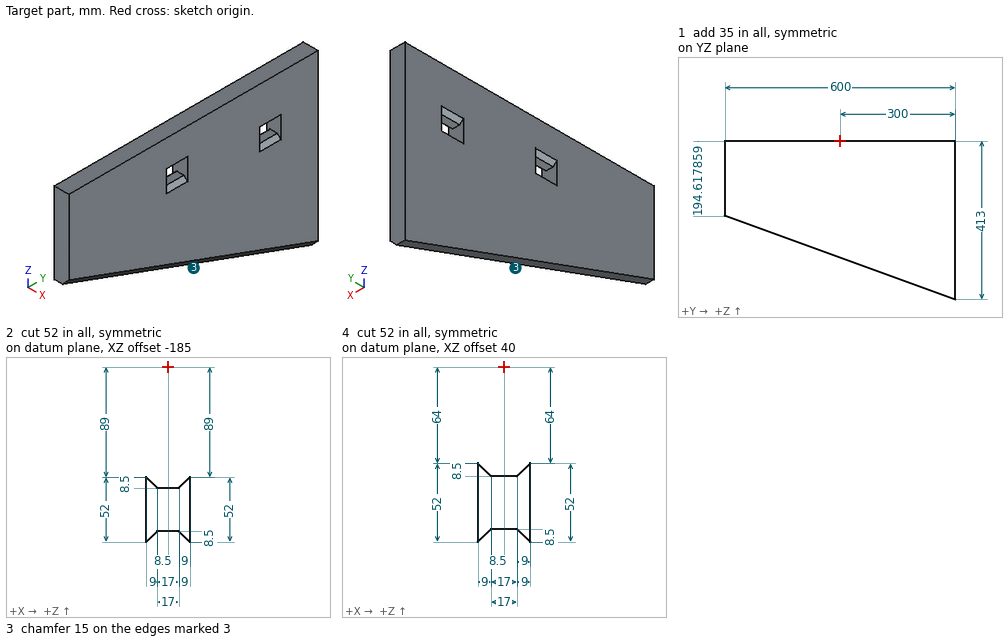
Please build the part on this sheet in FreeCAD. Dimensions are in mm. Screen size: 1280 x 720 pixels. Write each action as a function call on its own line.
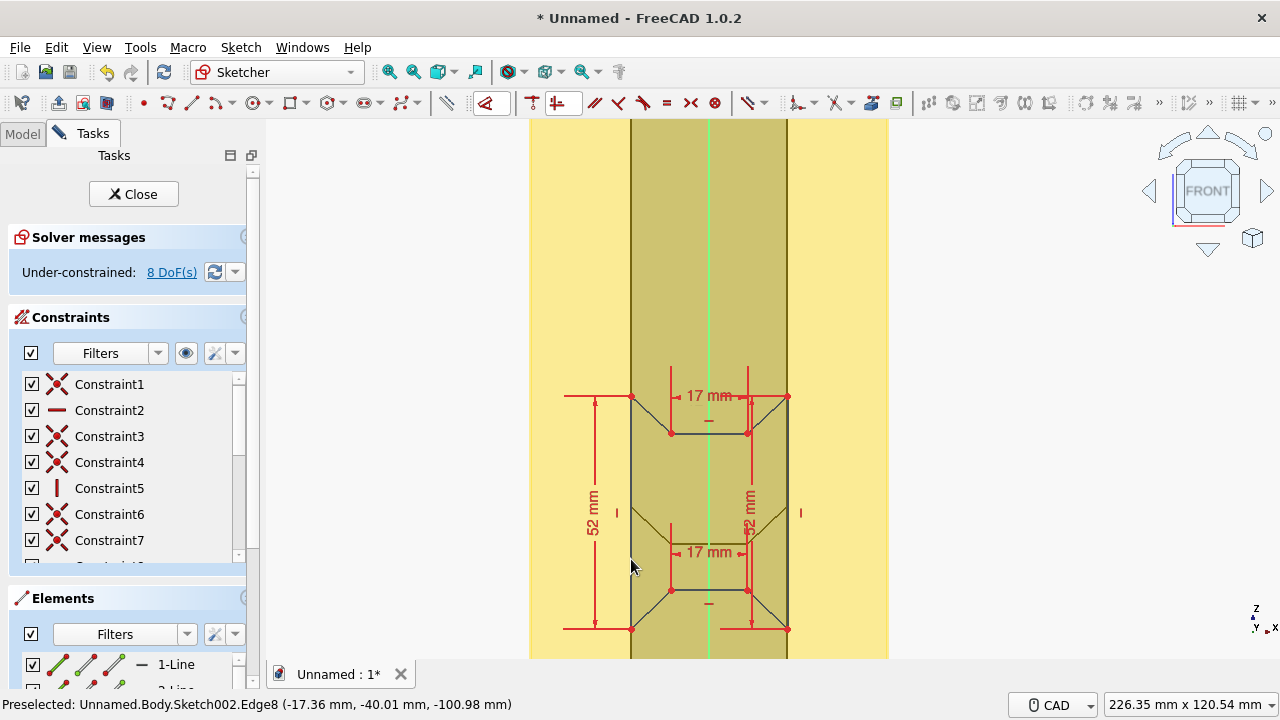
click(643, 408)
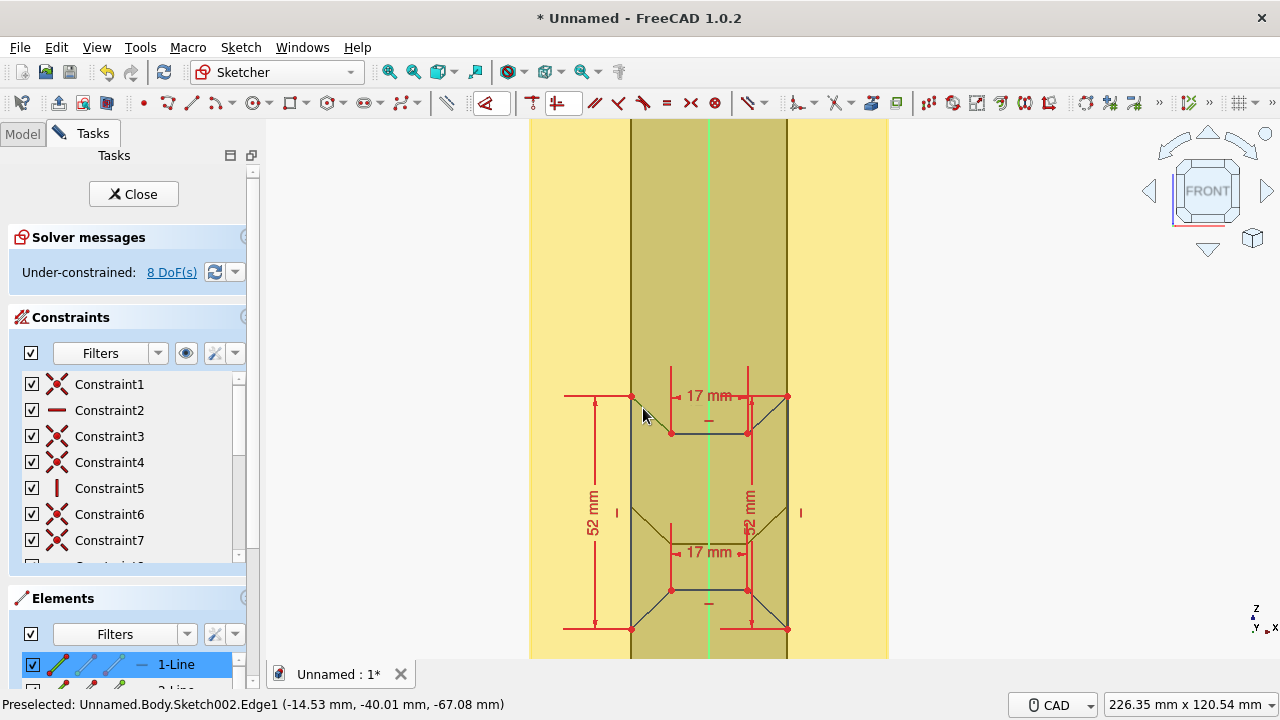
key(l)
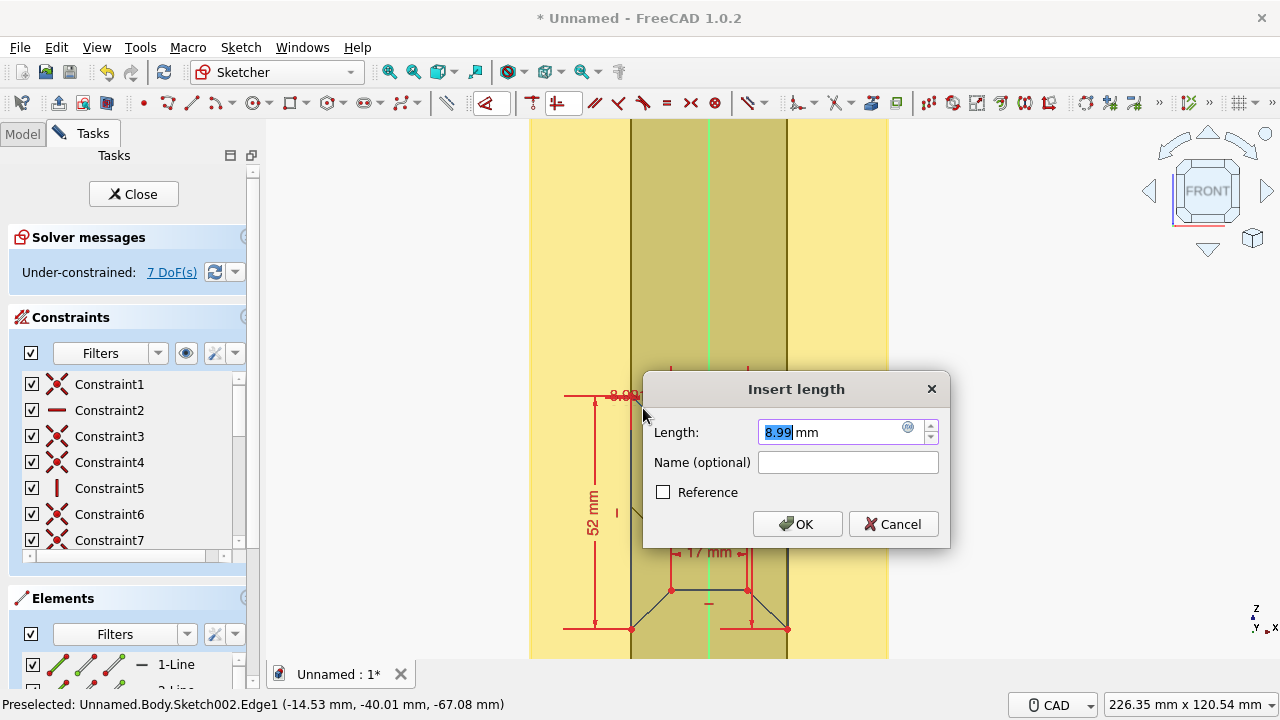
text(9)
key(Return)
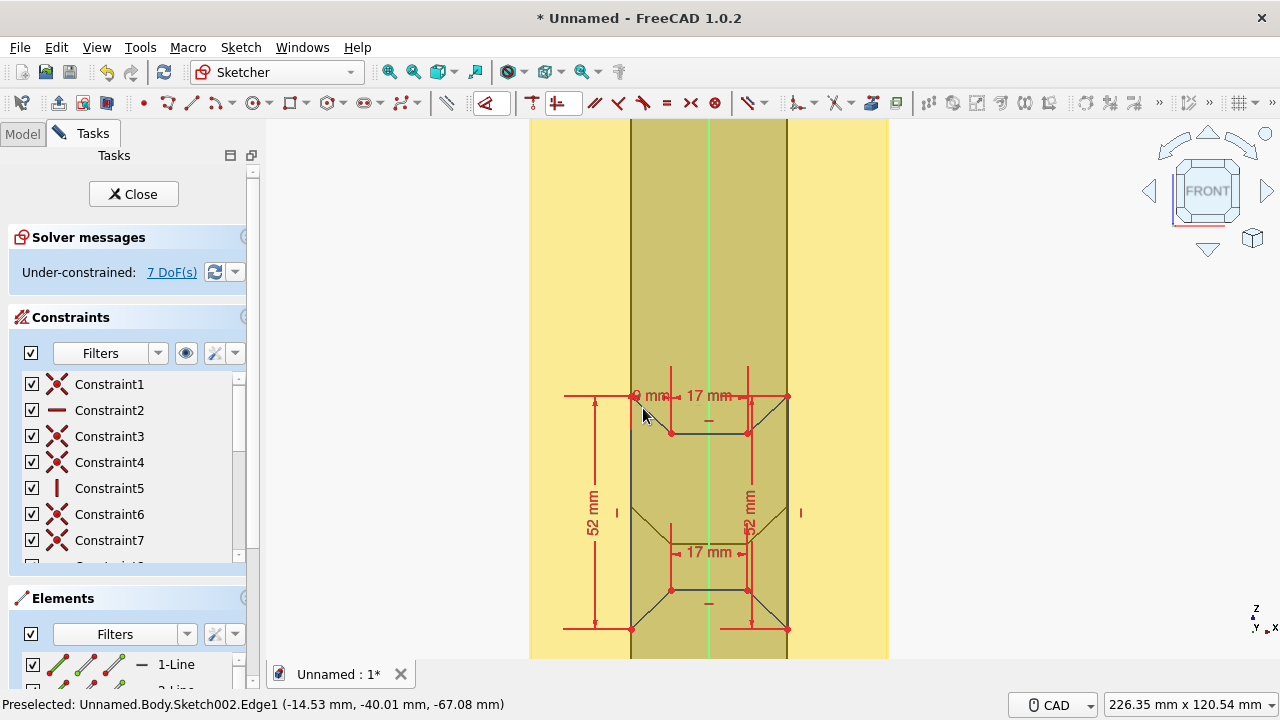
click(760, 422)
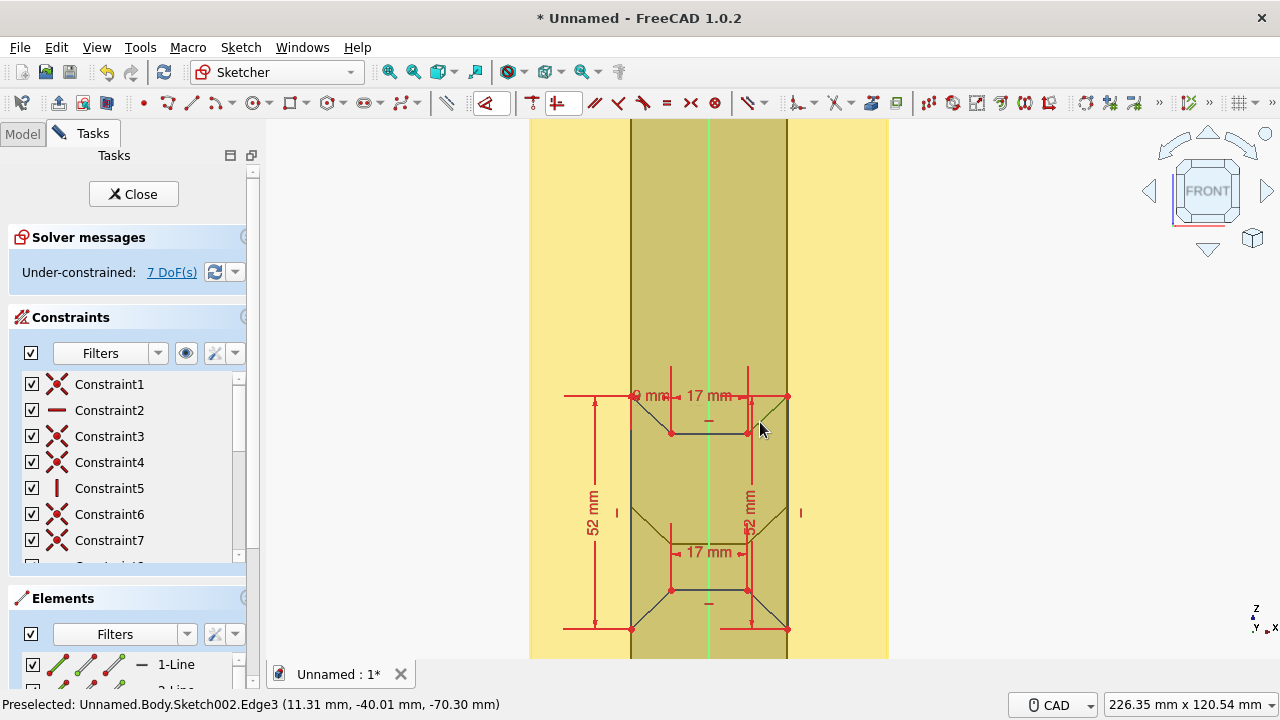
click(504, 104)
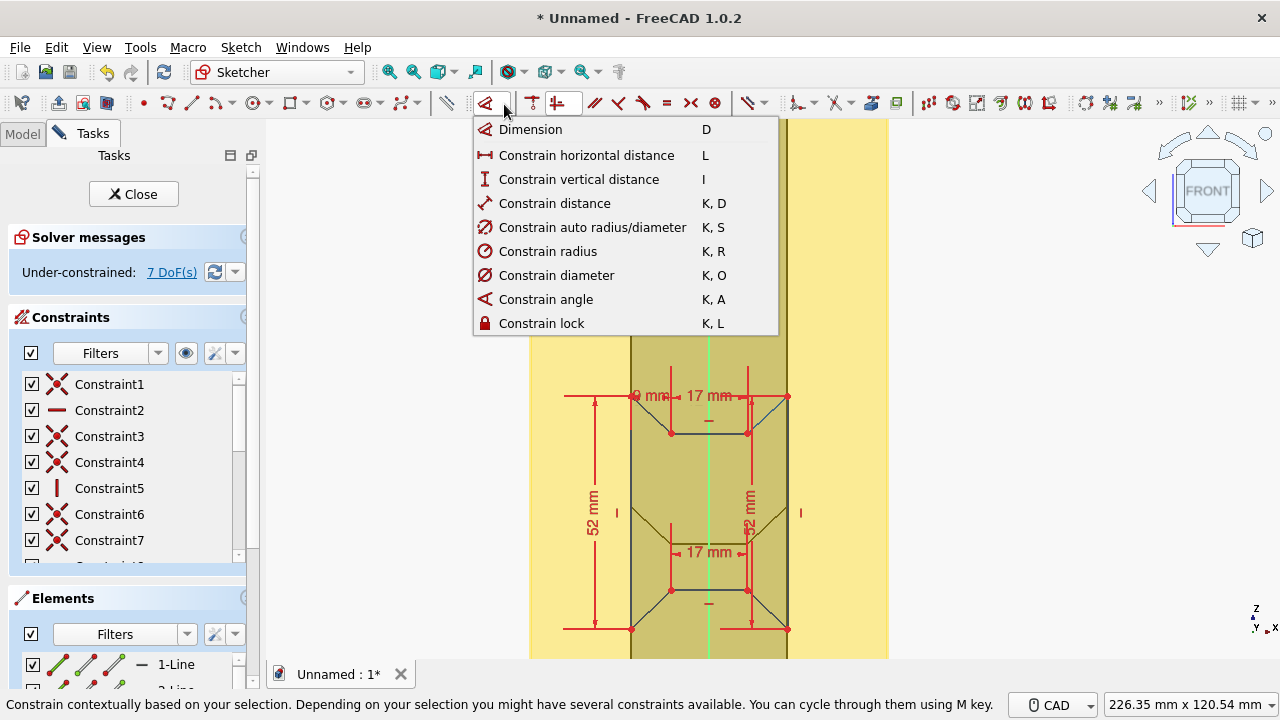
click(626, 155)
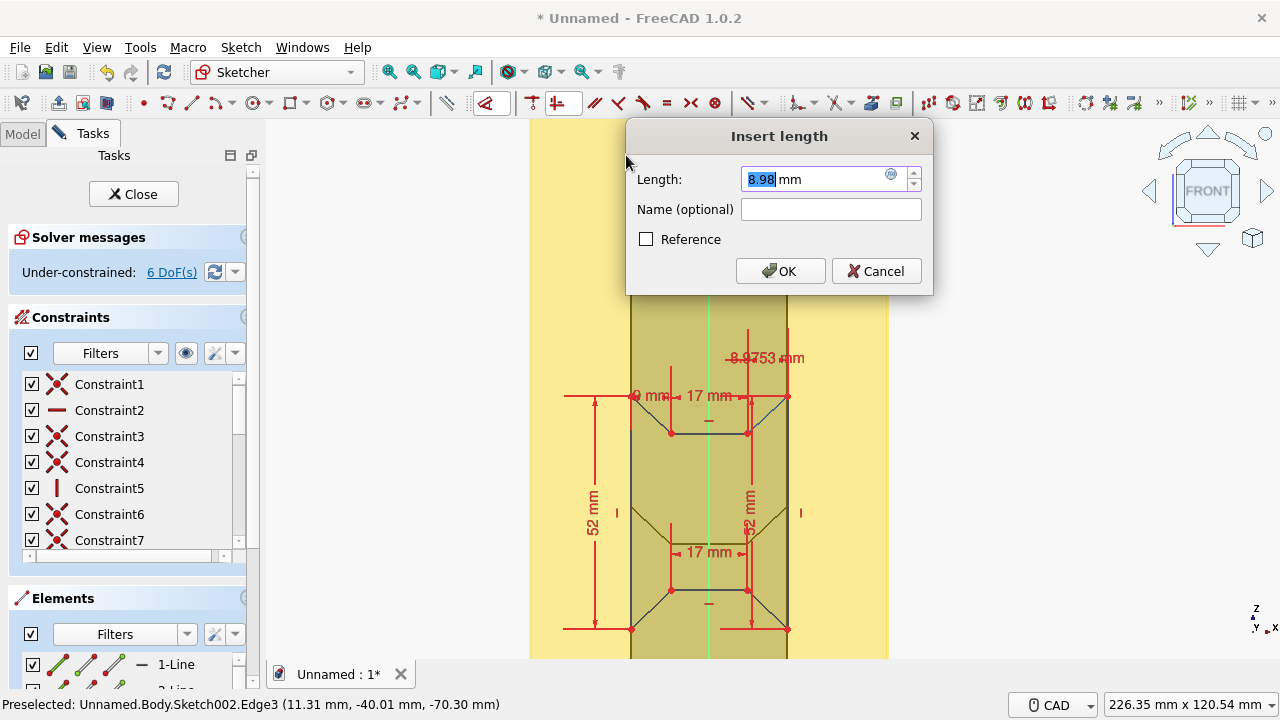
text(9)
key(Return)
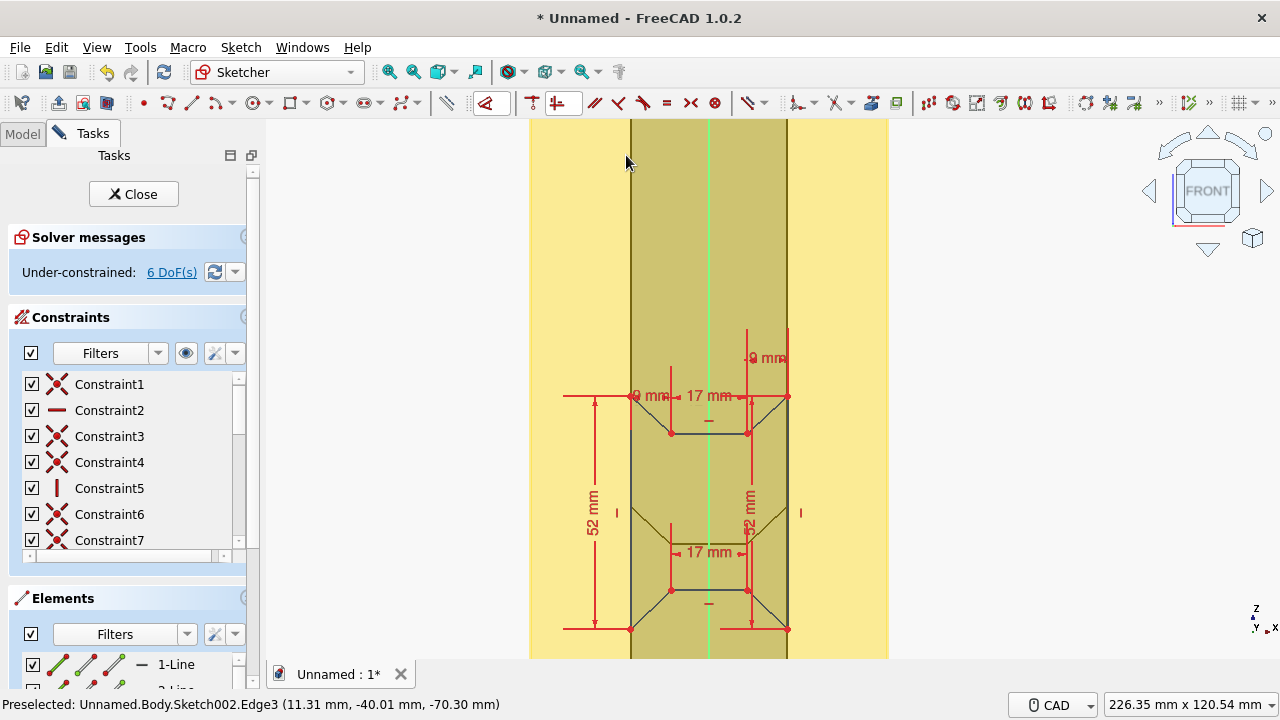
click(776, 618)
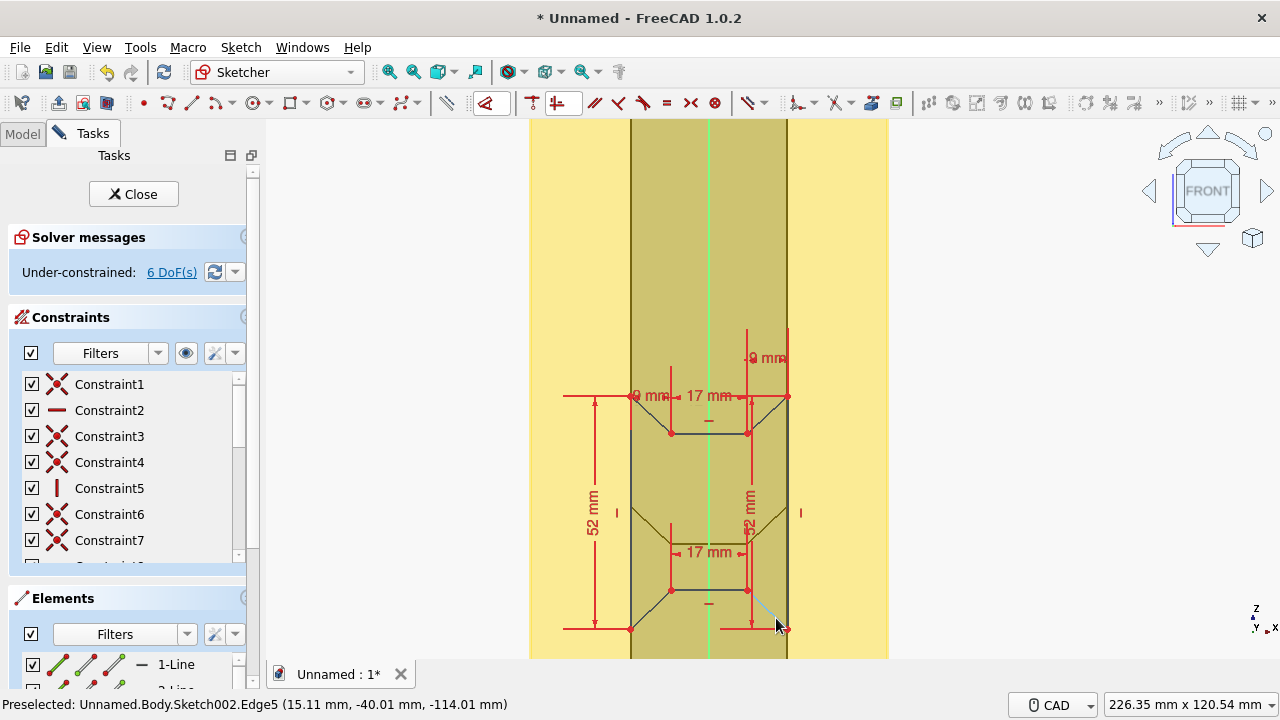
key(l)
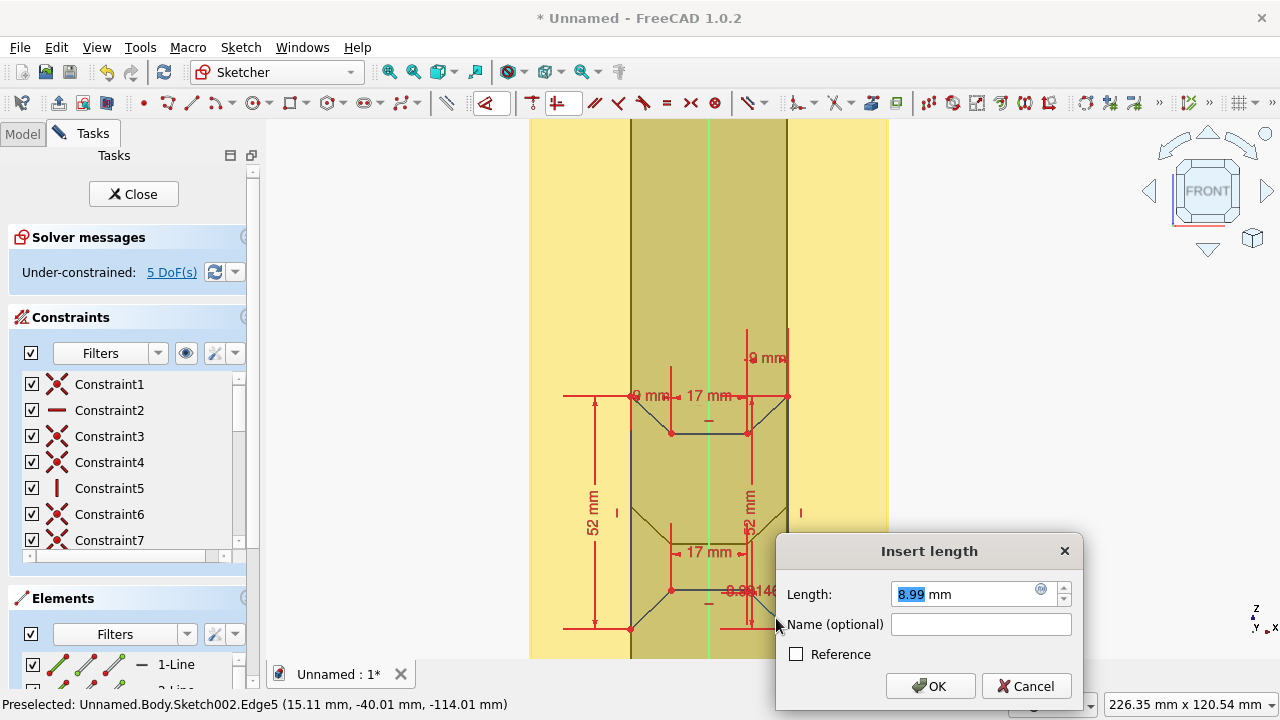
text(9)
key(Return)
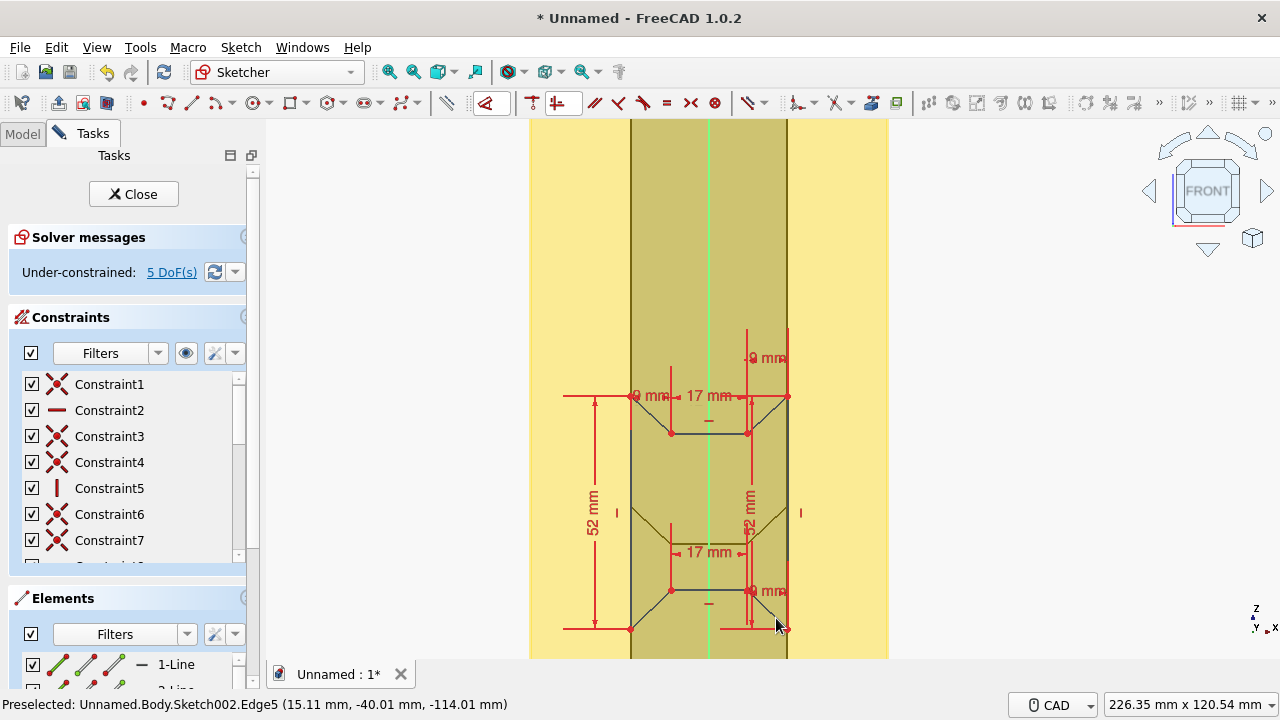
click(631, 396)